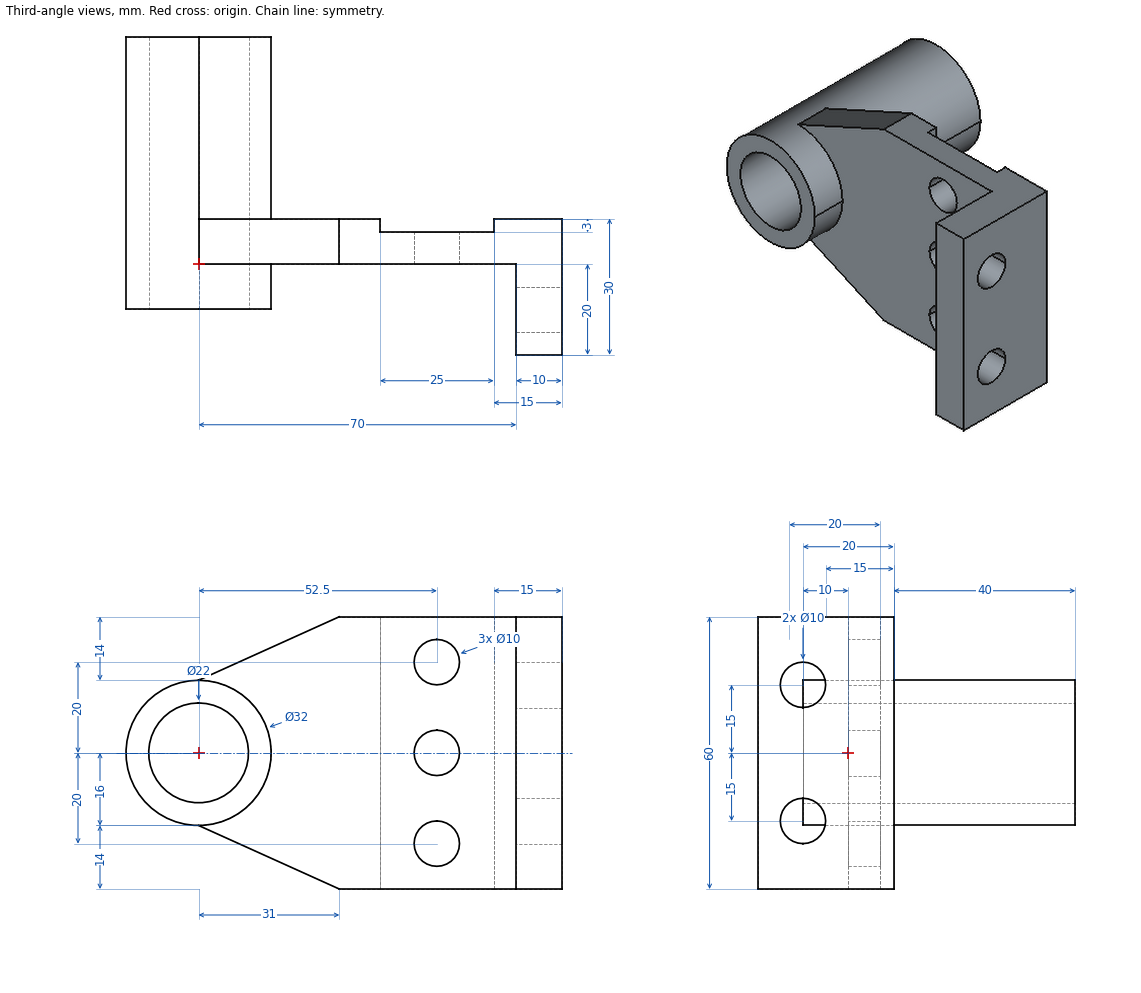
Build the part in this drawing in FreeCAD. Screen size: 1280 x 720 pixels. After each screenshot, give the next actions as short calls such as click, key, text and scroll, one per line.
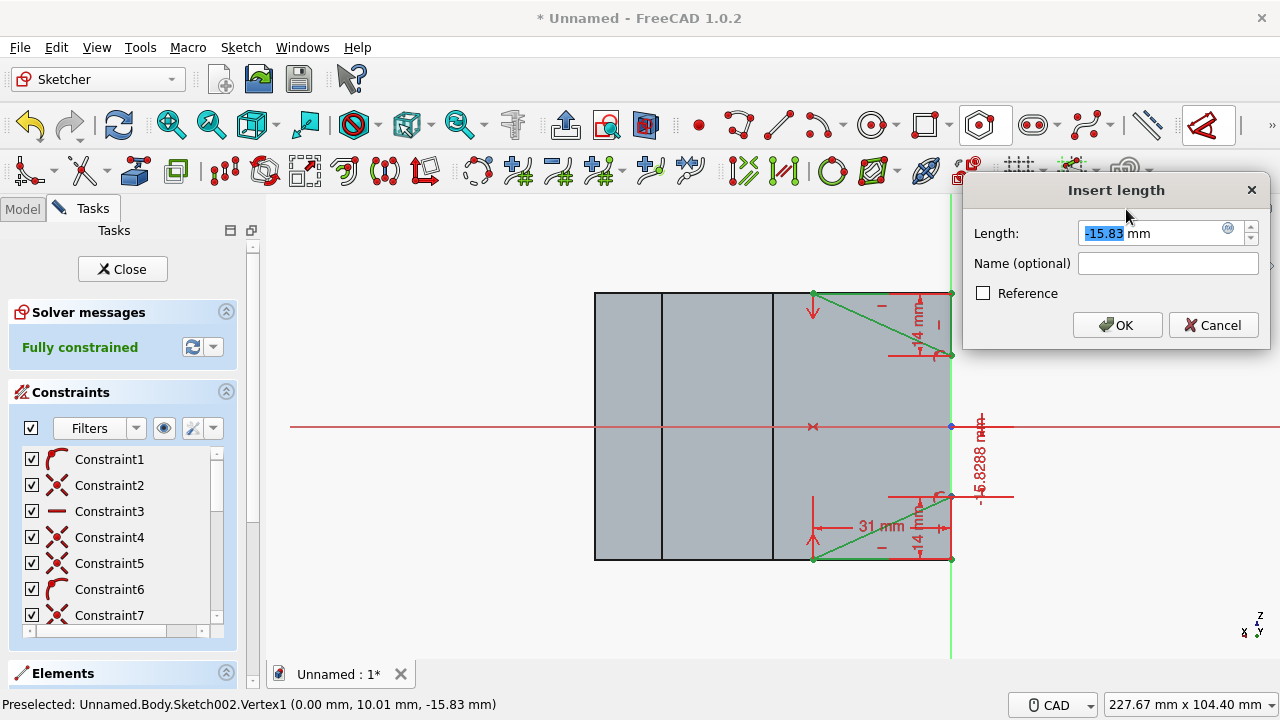
text(-16)
key(Return)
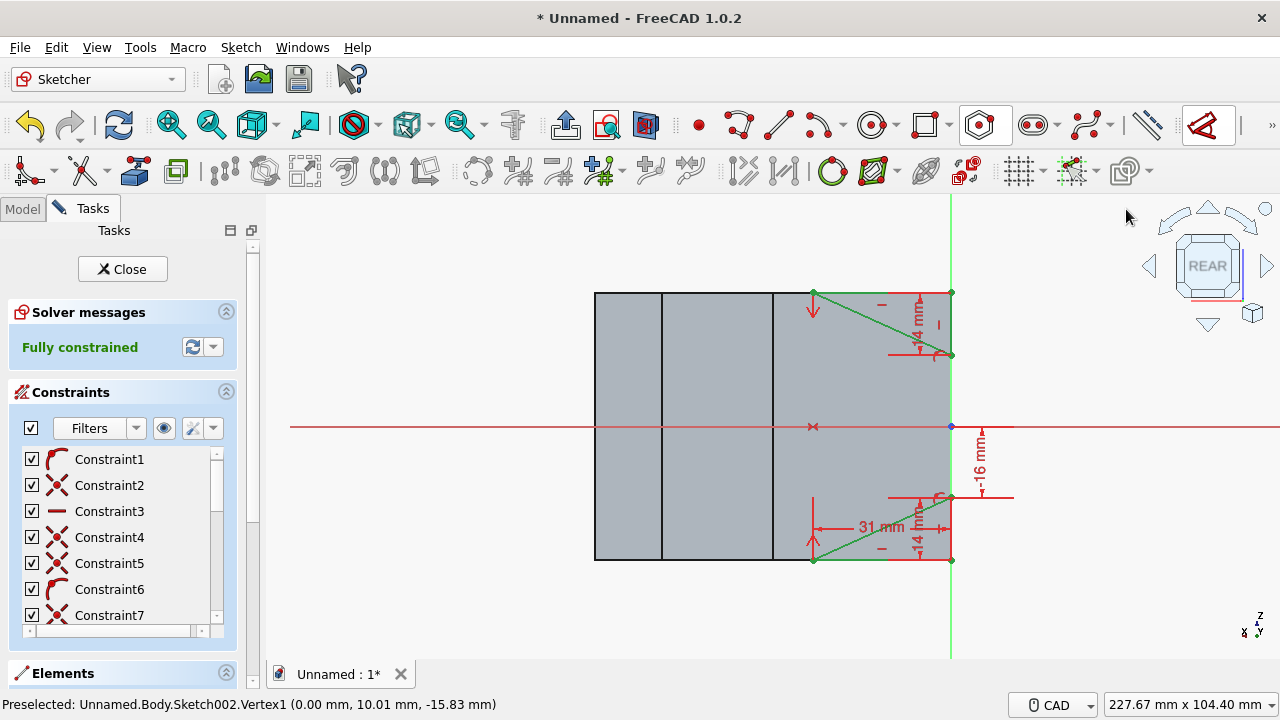
click(123, 269)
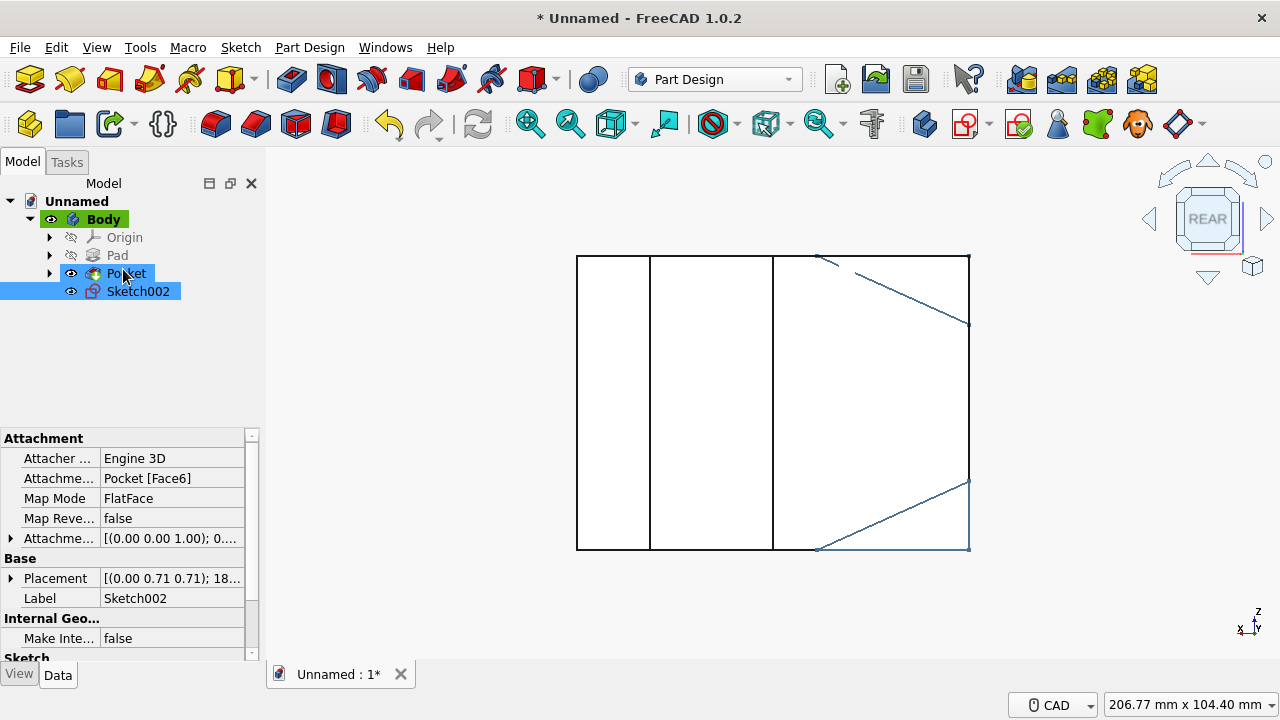
click(292, 80)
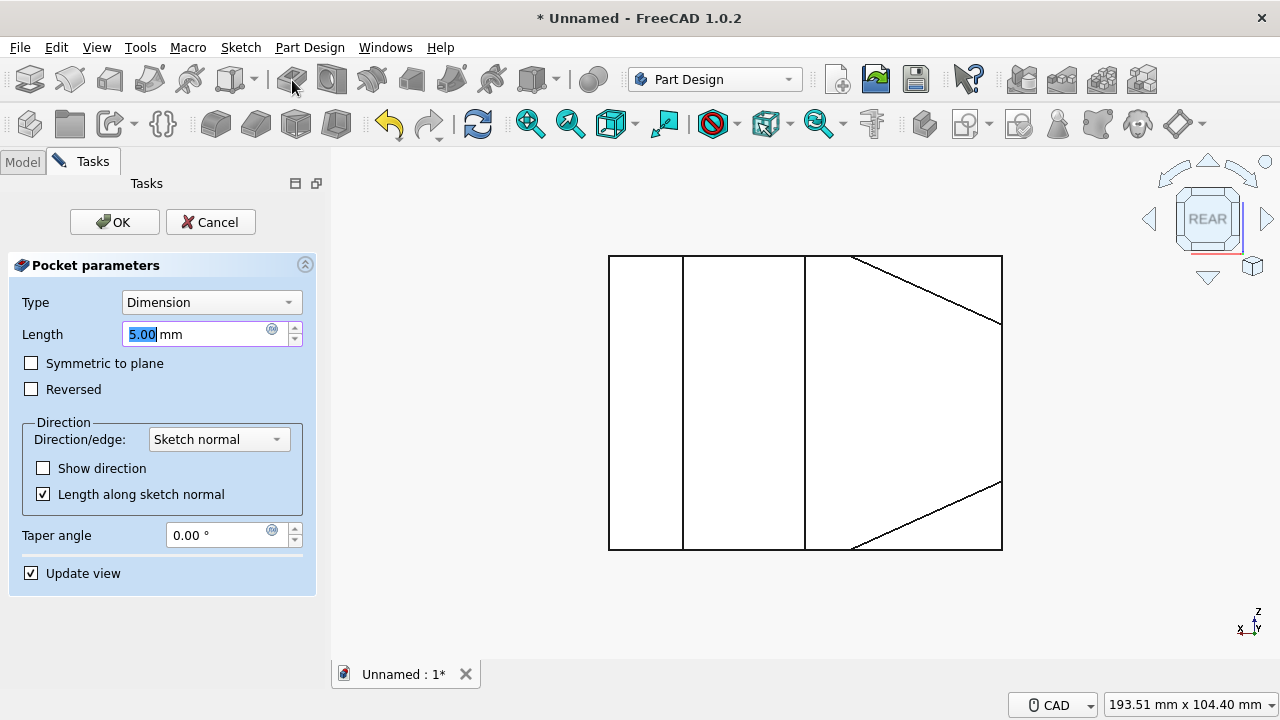
text(15)
key(Tab)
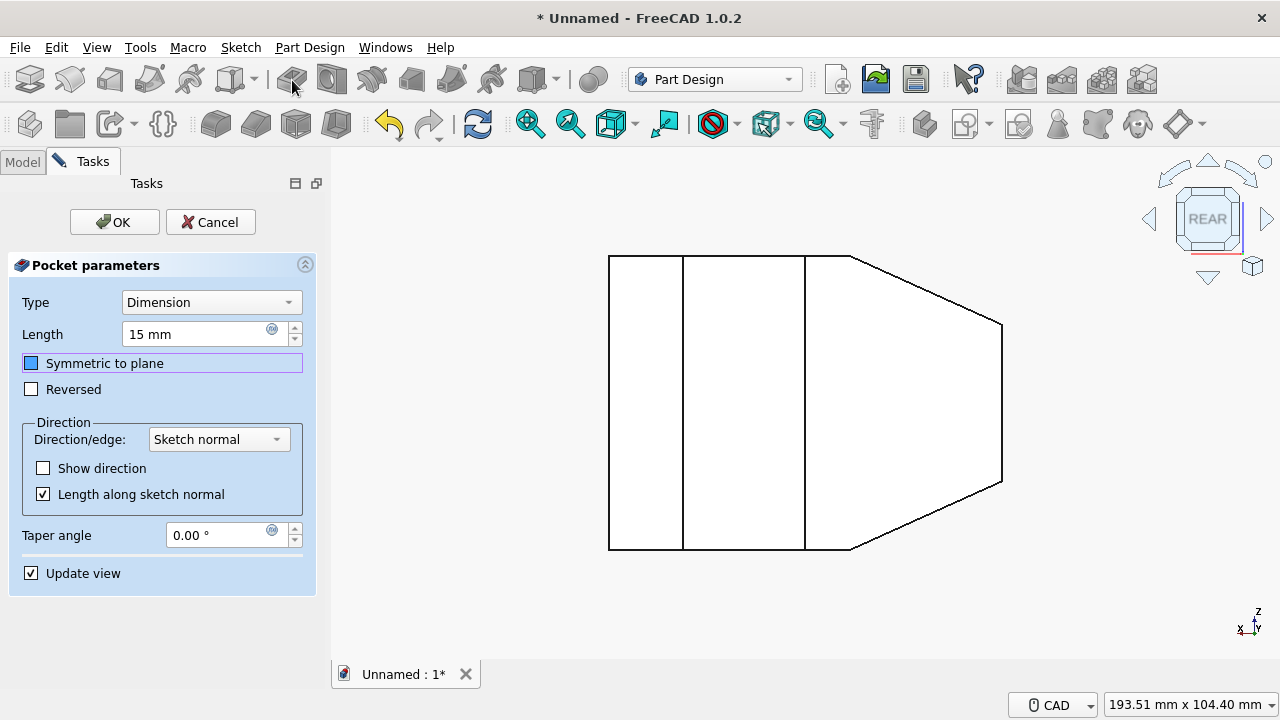
click(115, 222)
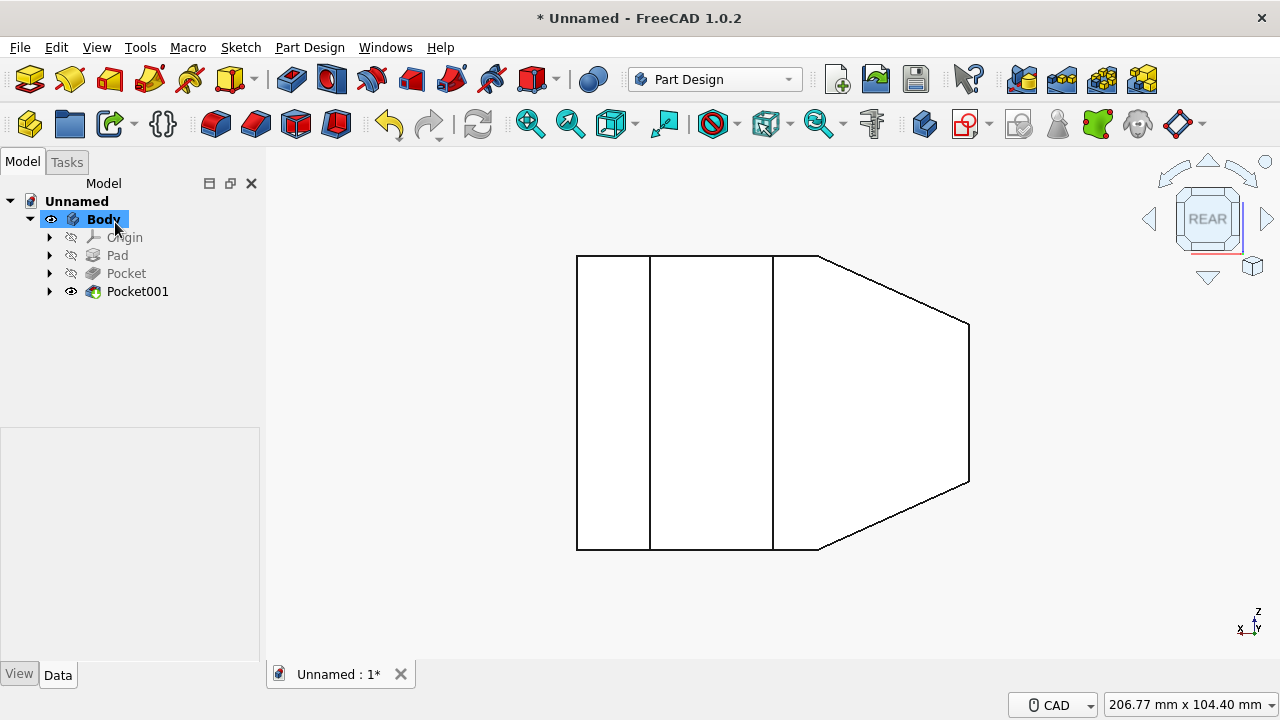
click(871, 402)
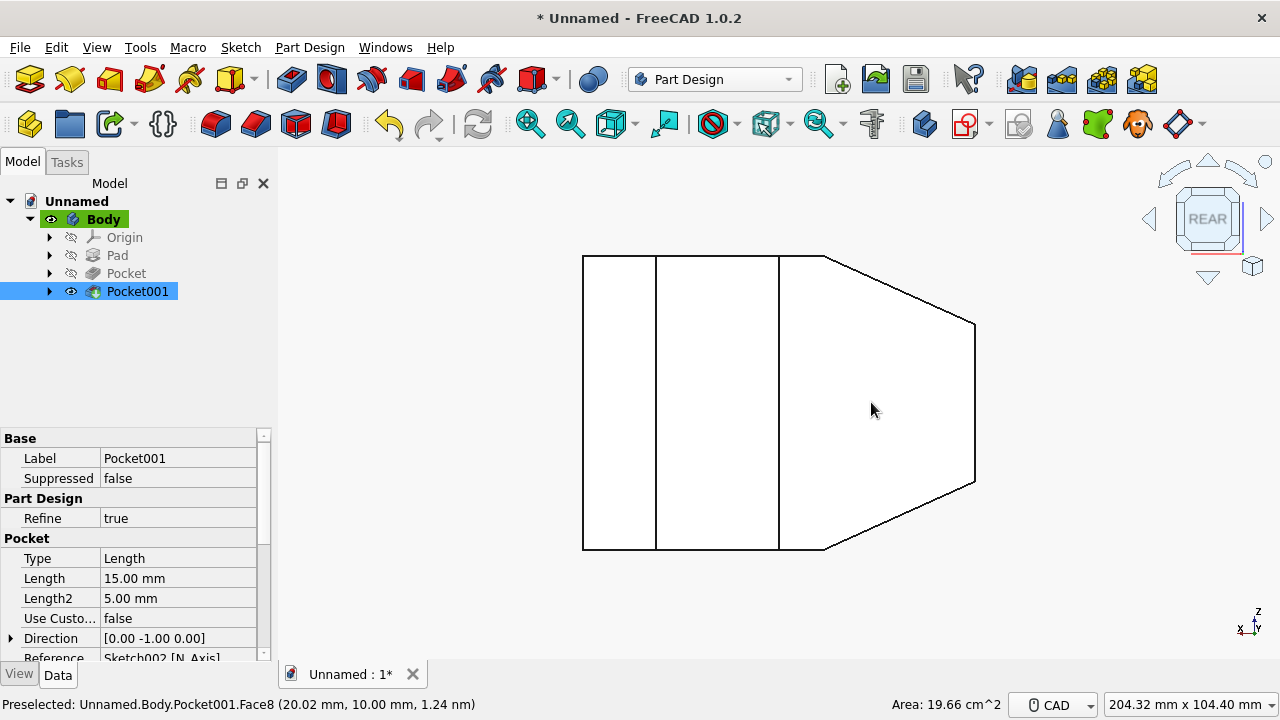
click(966, 124)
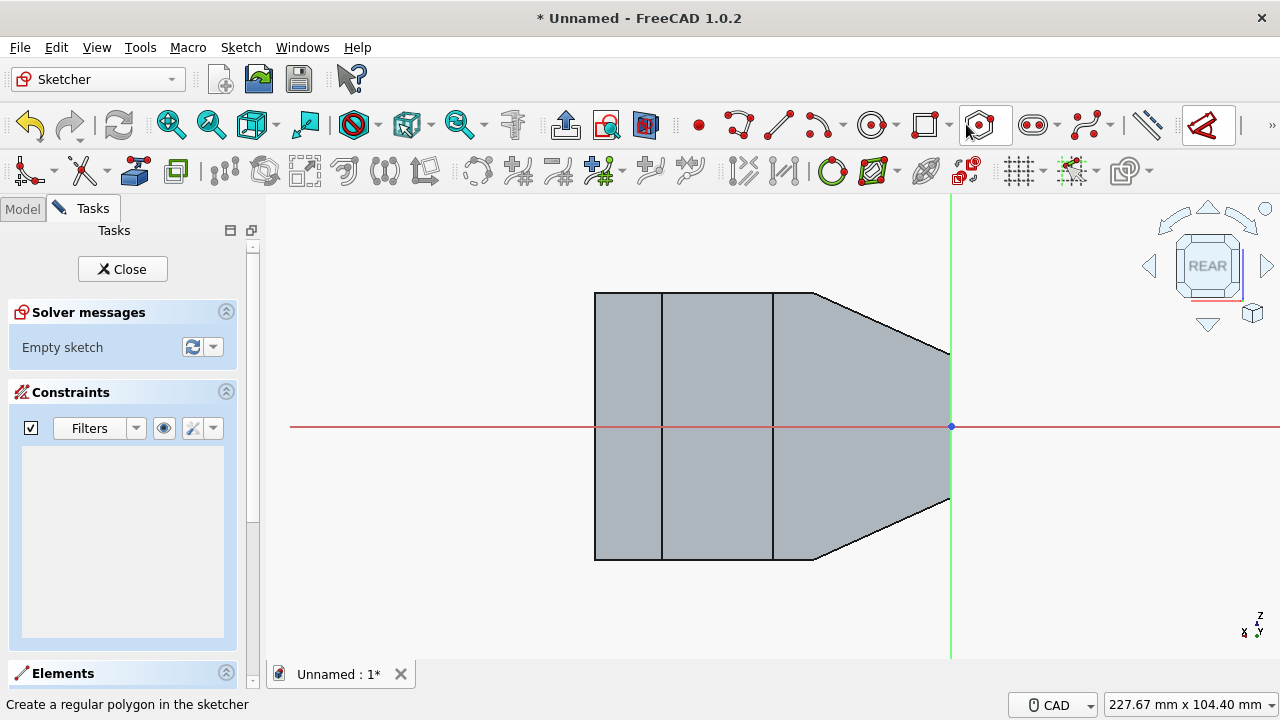
scroll(1115, 427, up, 4)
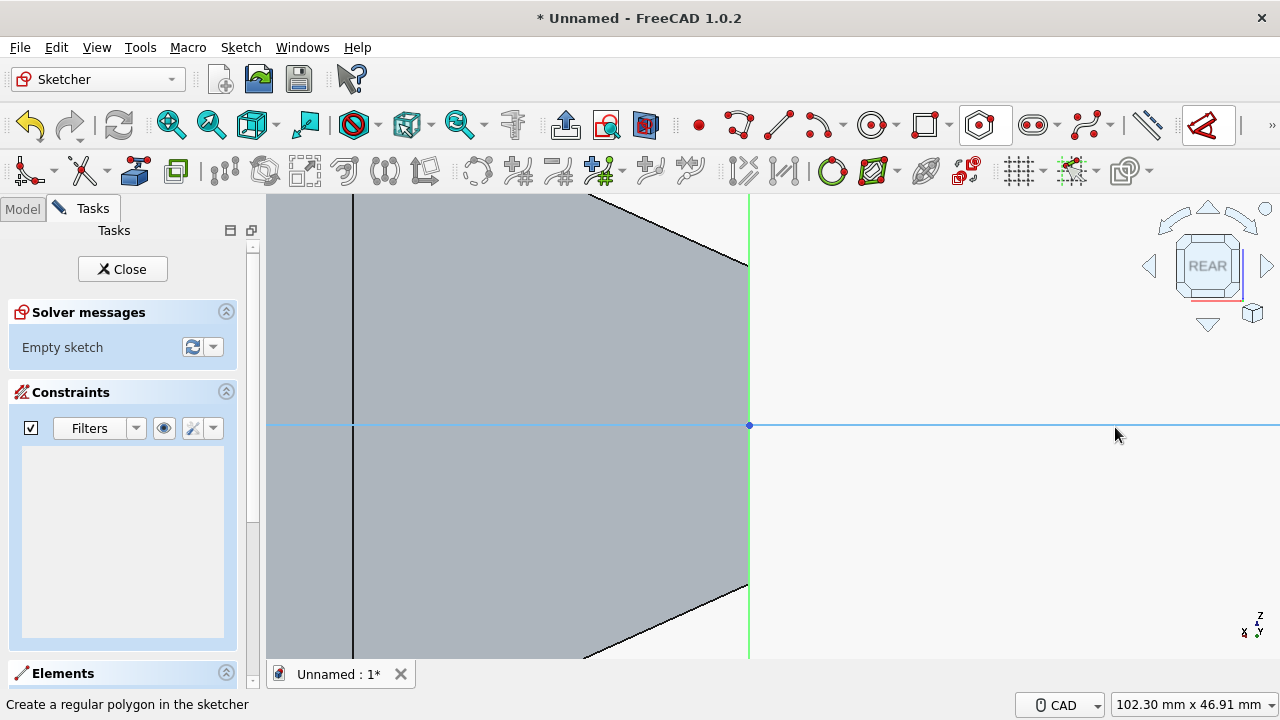
click(872, 126)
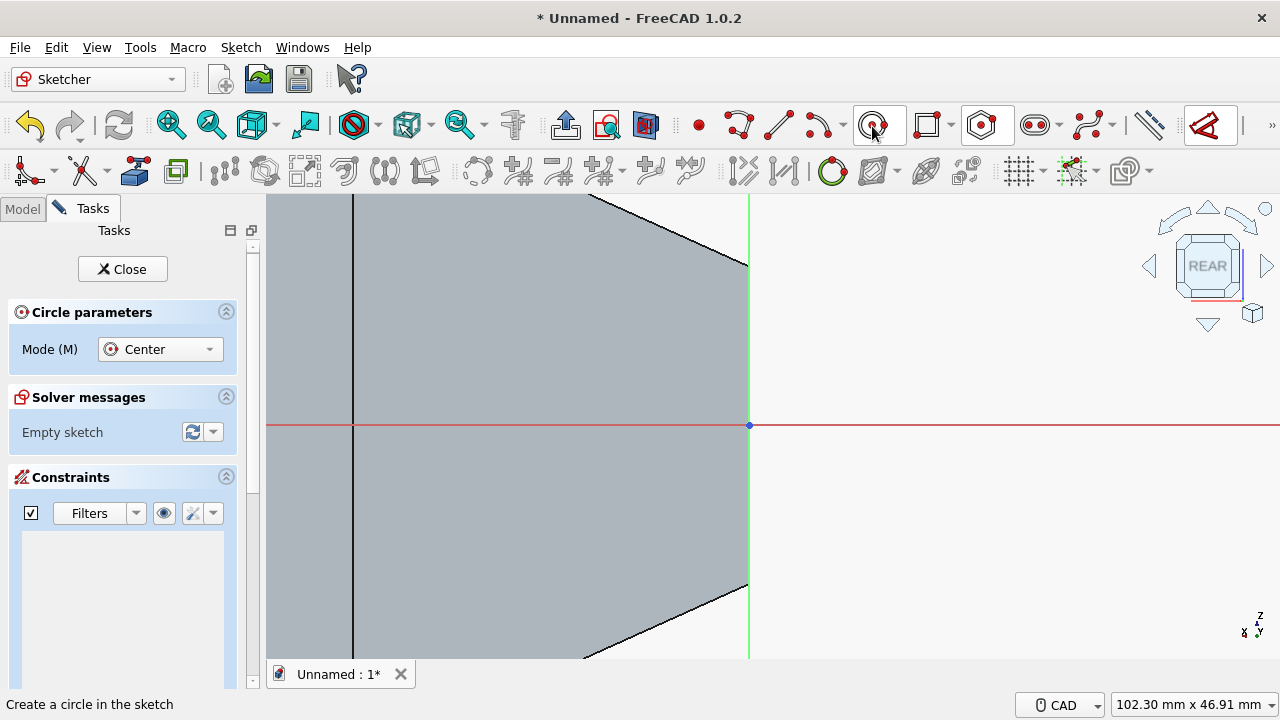
click(749, 425)
move(861, 313)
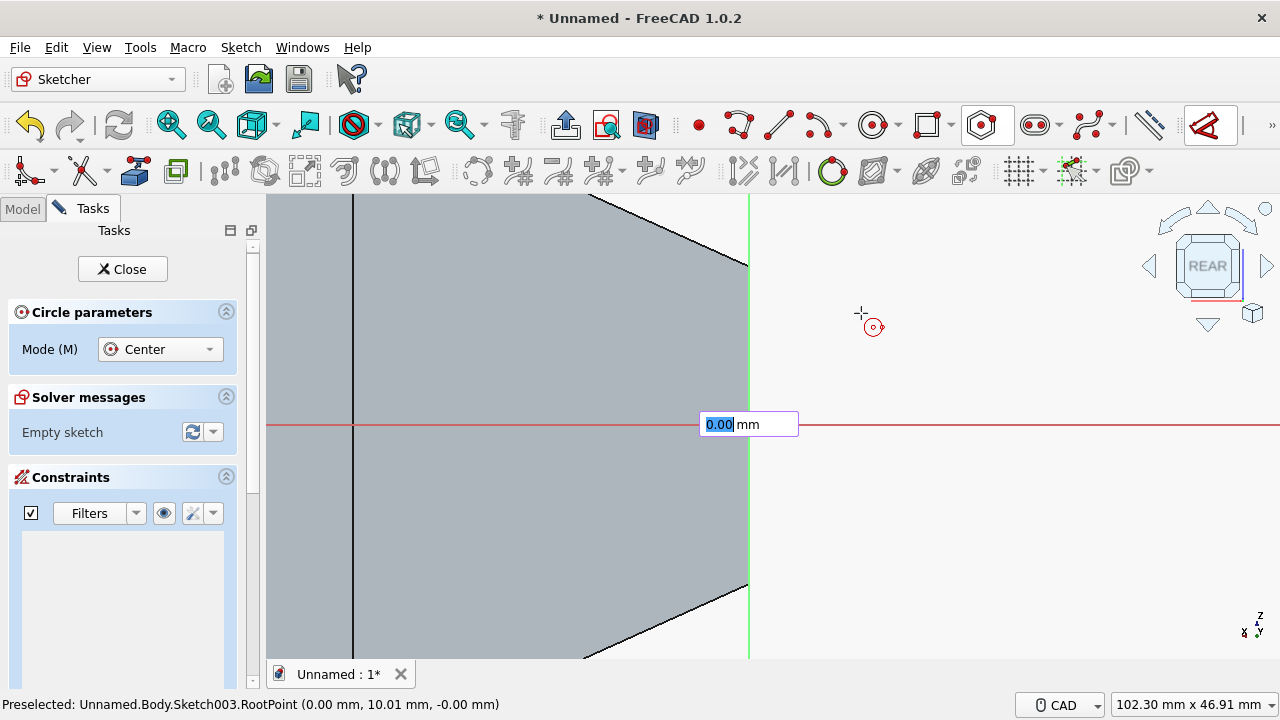
text(32)
key(Return)